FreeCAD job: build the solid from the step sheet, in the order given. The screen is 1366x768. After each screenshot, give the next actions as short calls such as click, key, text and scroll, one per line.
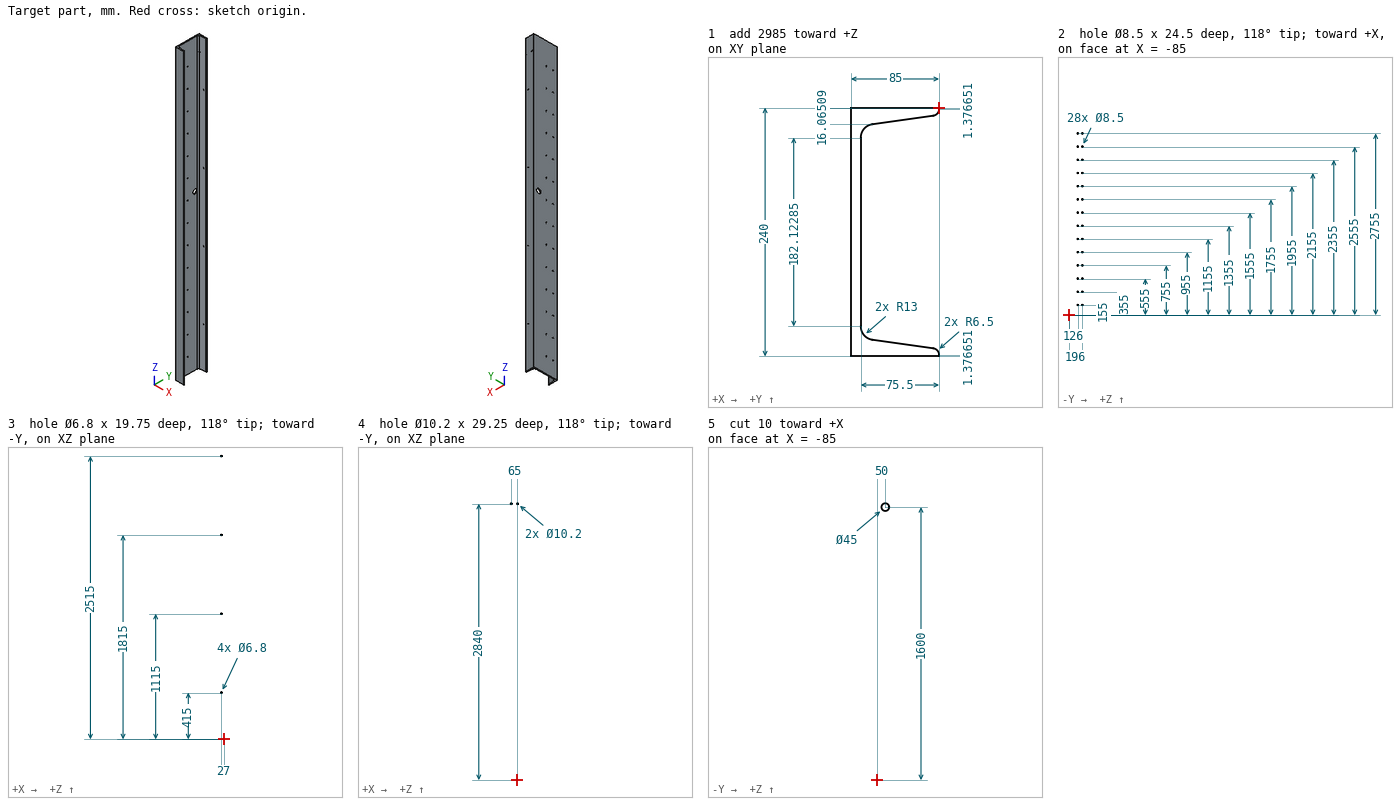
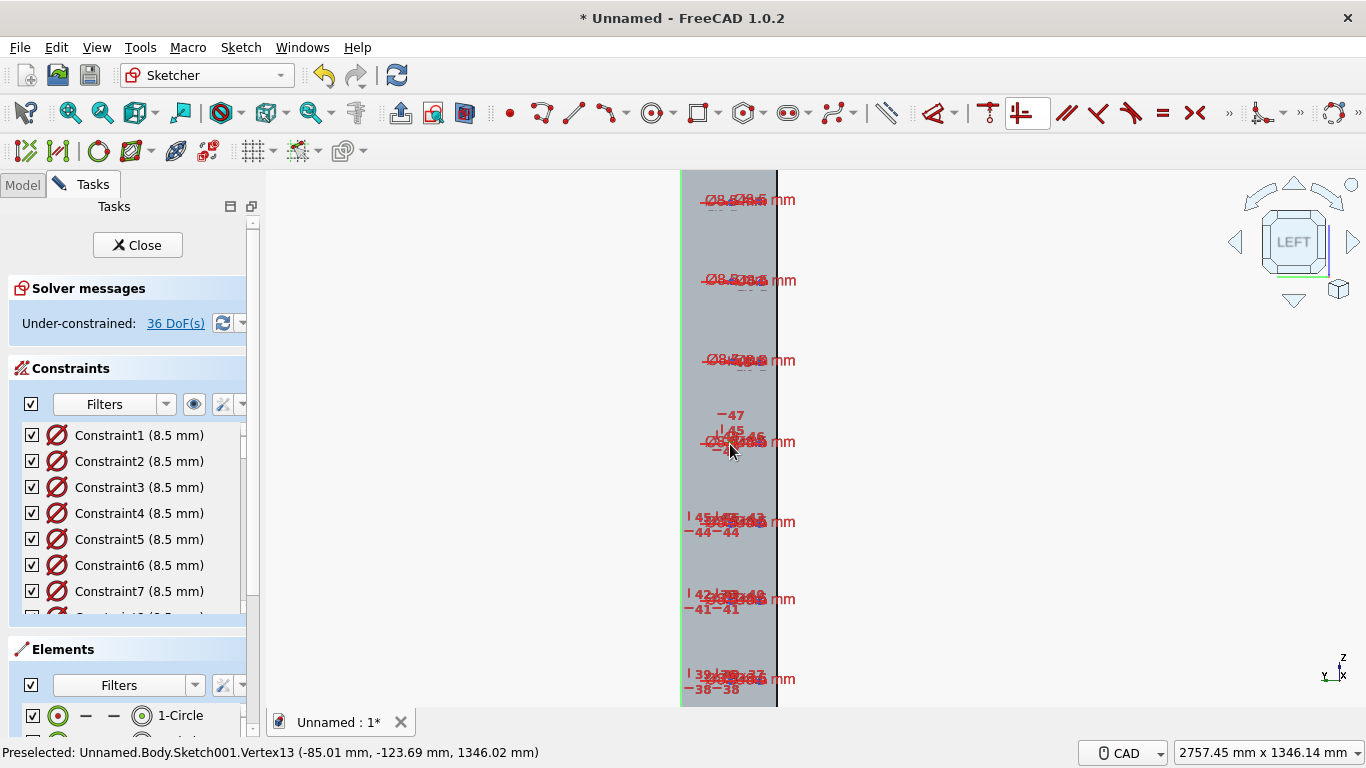
scroll(732, 362, up, 4)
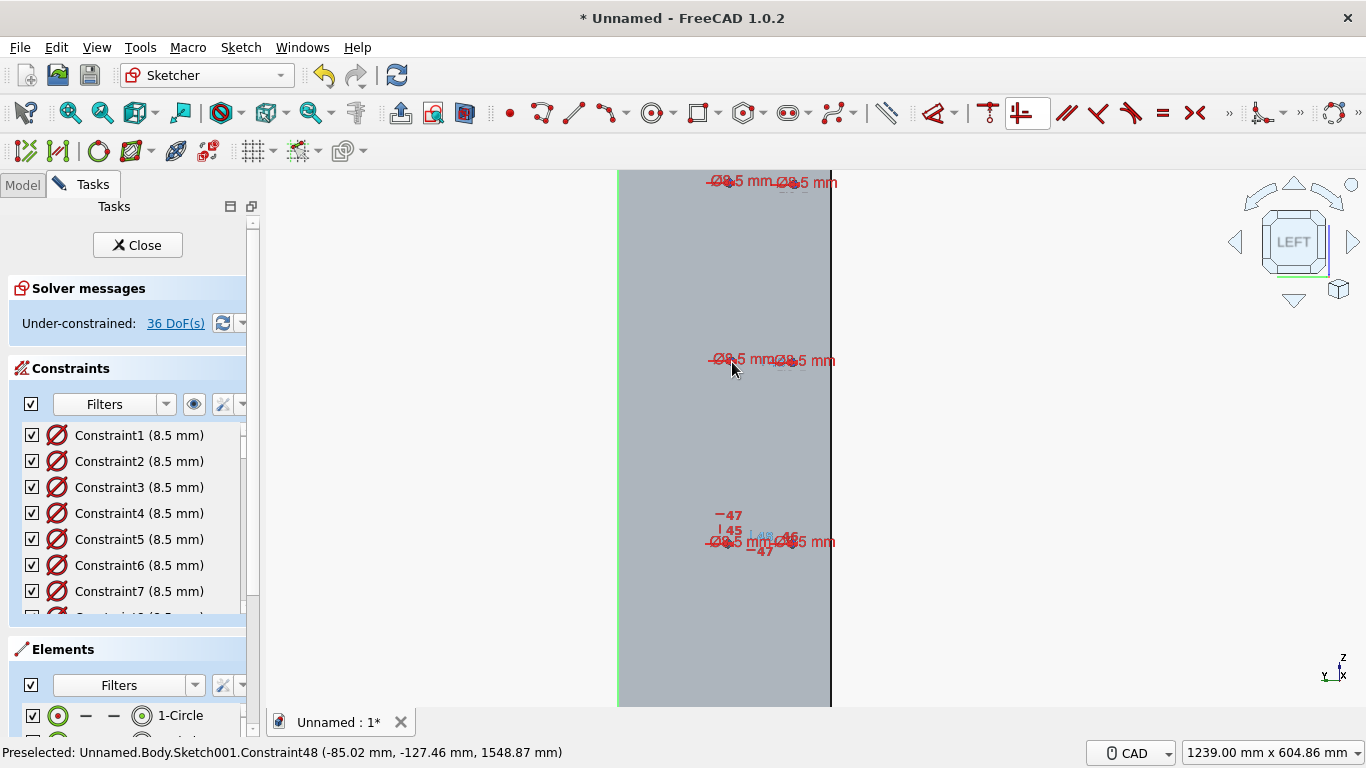
click(732, 361)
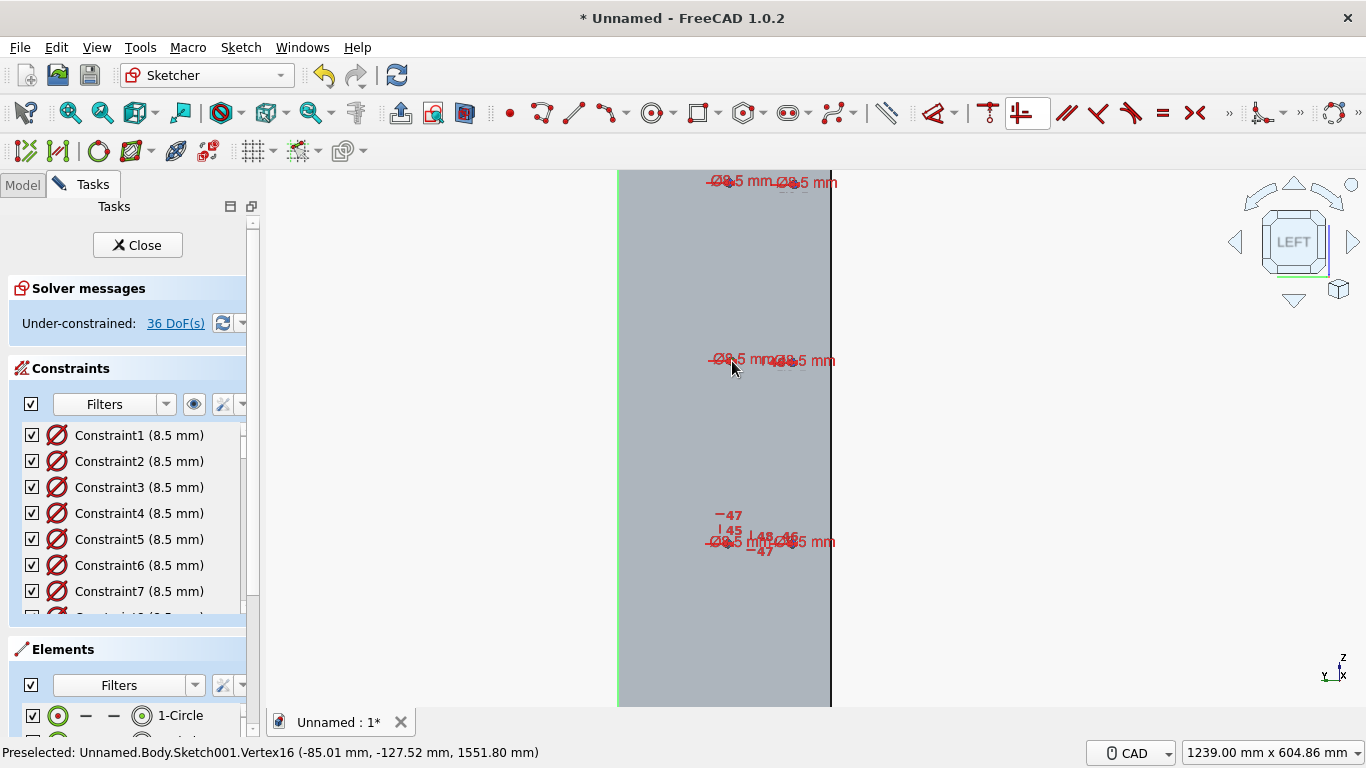
click(1044, 114)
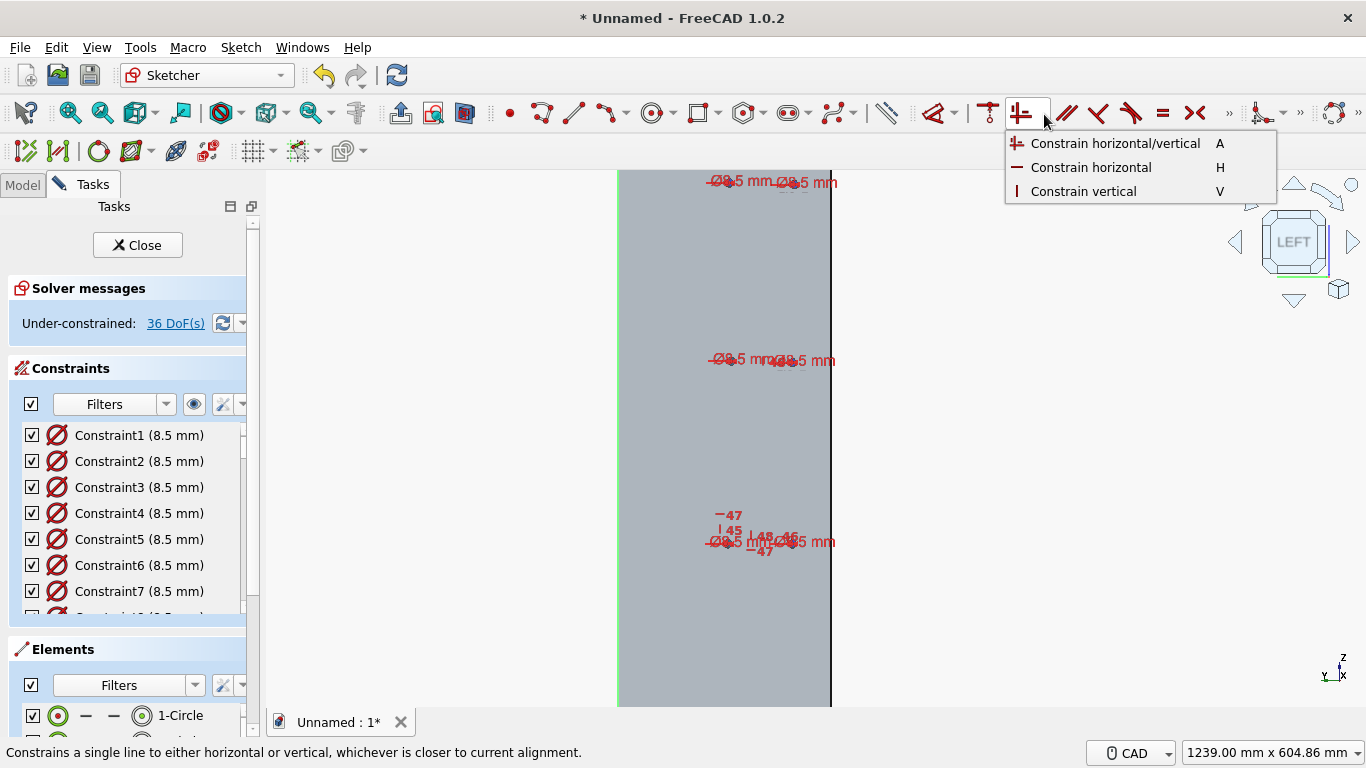
click(1141, 191)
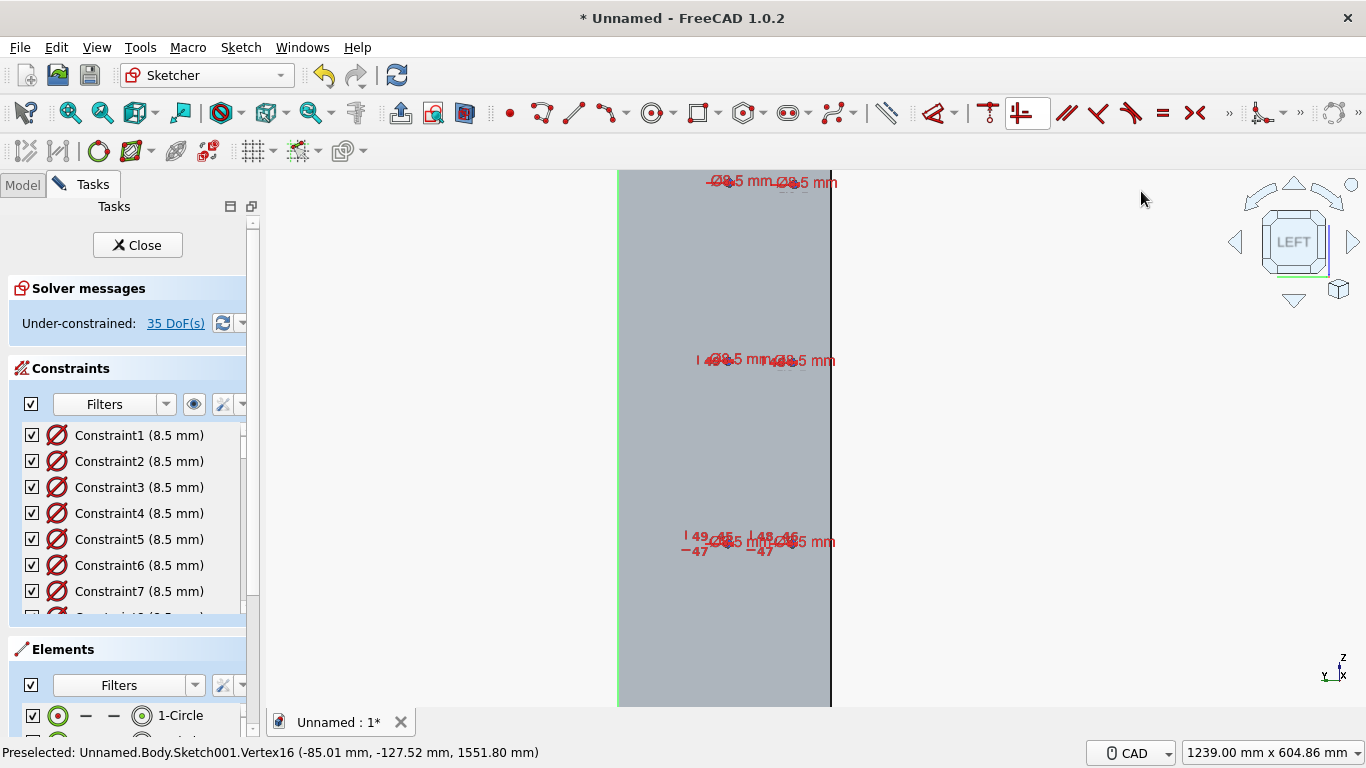
scroll(754, 427, down, 10)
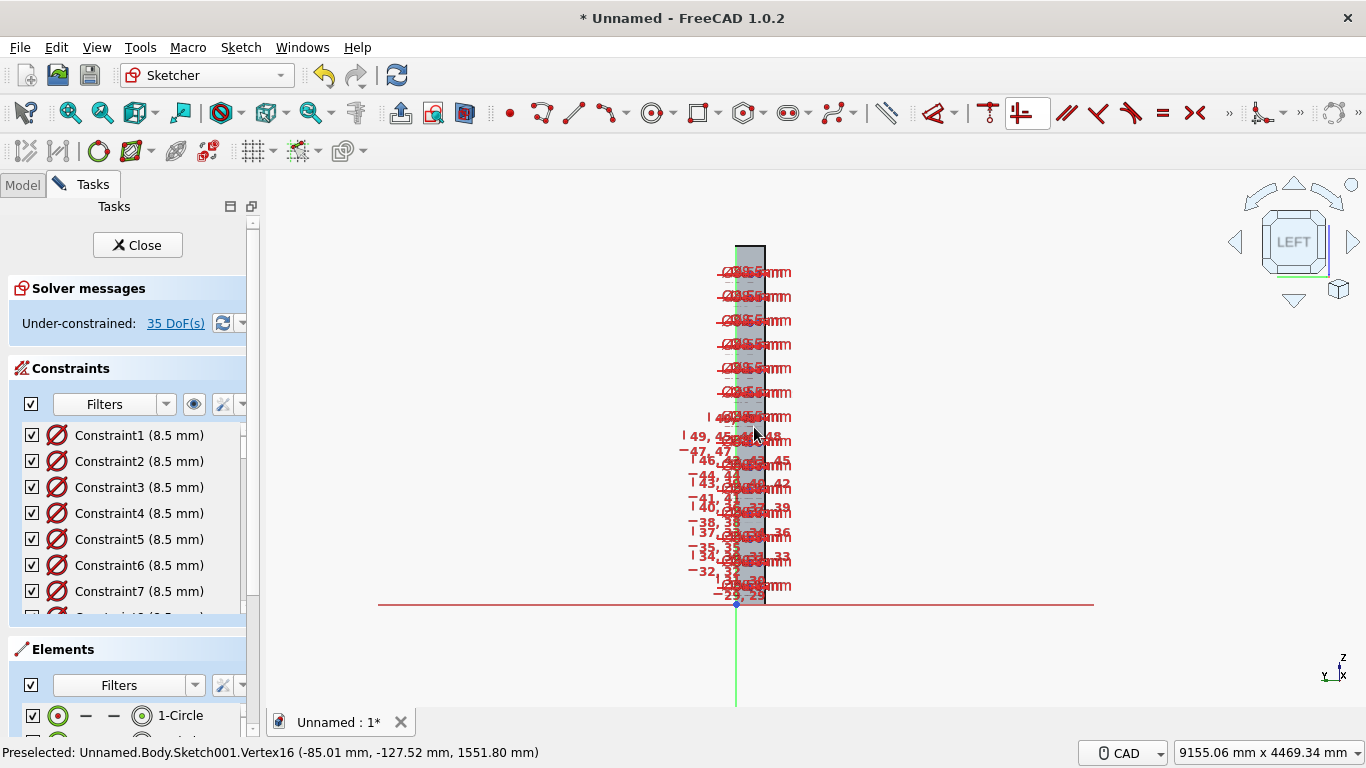
scroll(760, 419, up, 2)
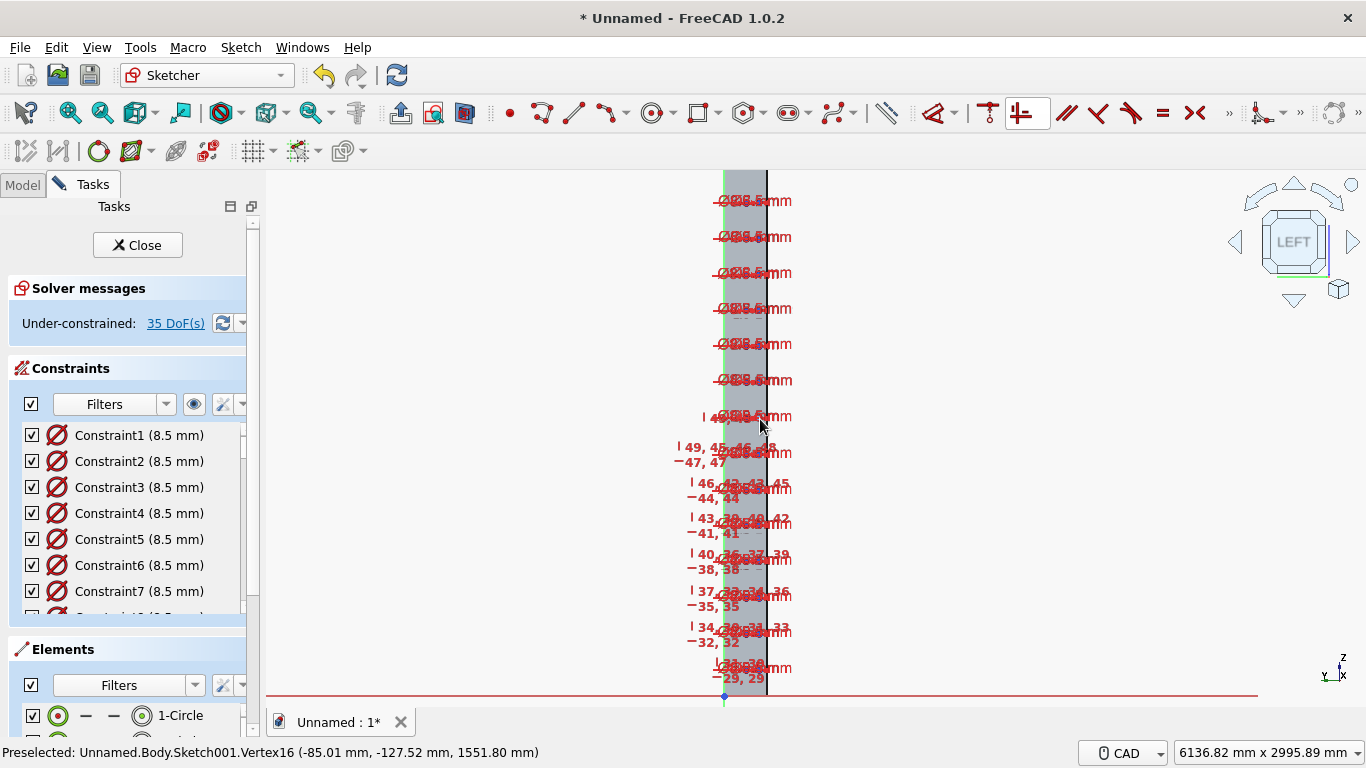
click(759, 418)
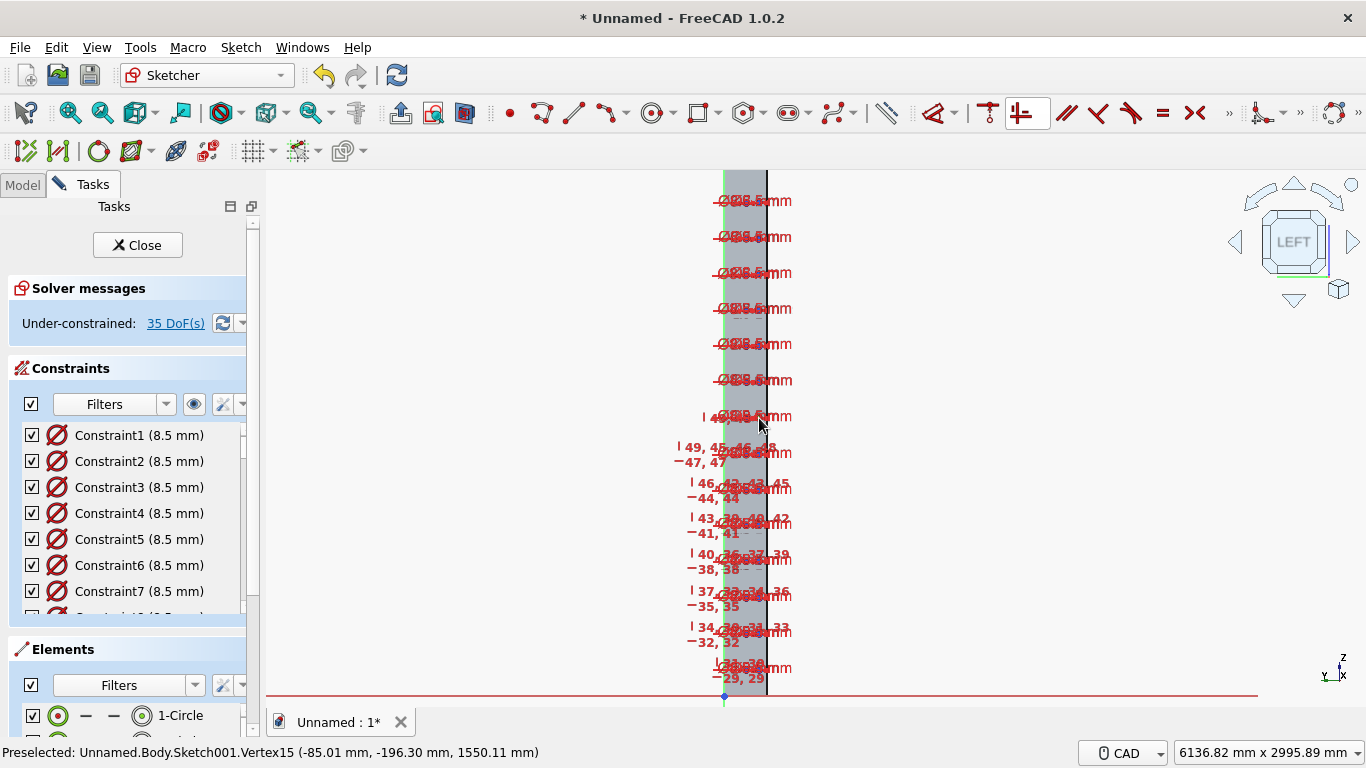
scroll(746, 418, up, 4)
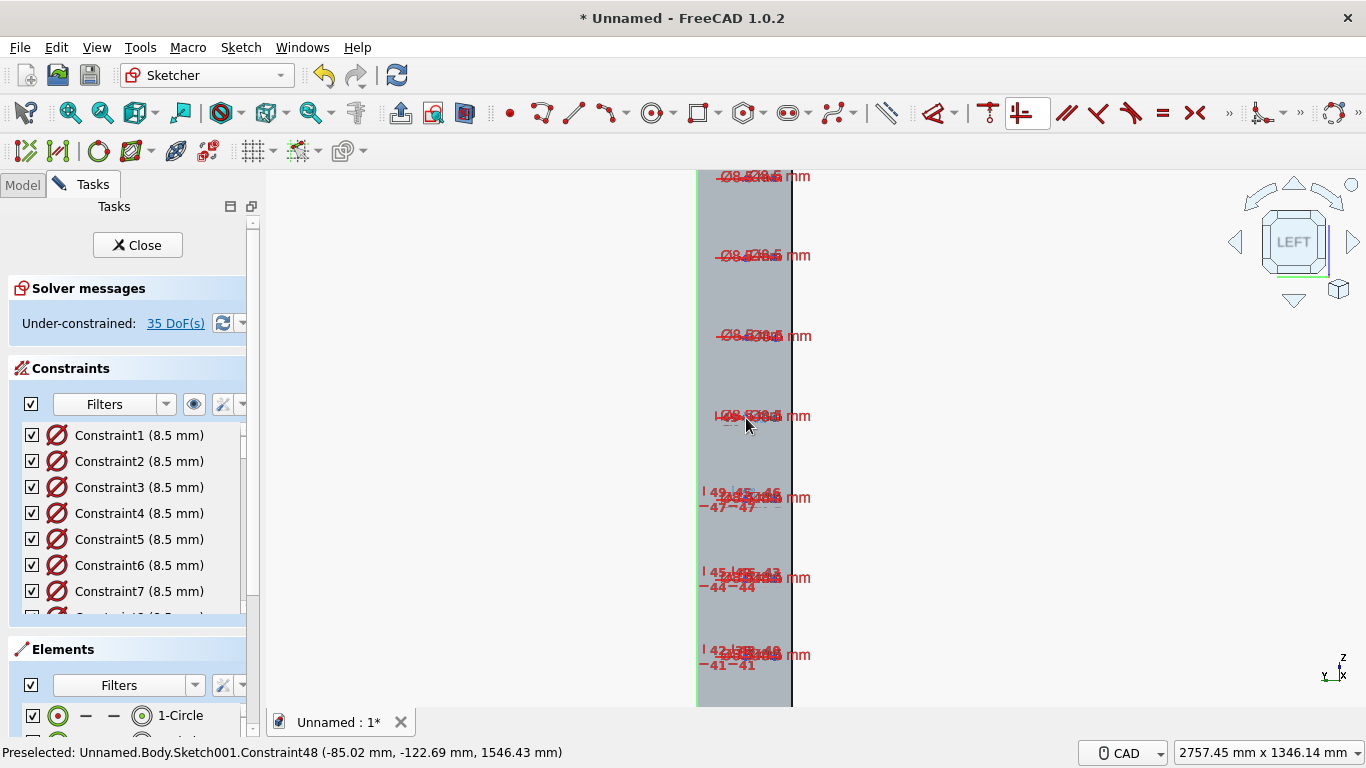
scroll(746, 418, up, 4)